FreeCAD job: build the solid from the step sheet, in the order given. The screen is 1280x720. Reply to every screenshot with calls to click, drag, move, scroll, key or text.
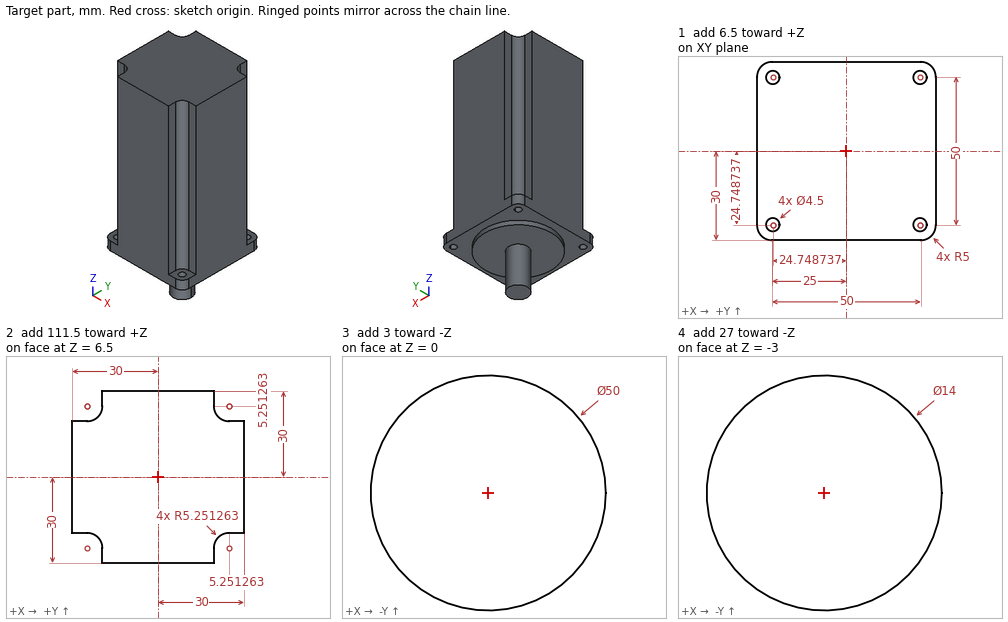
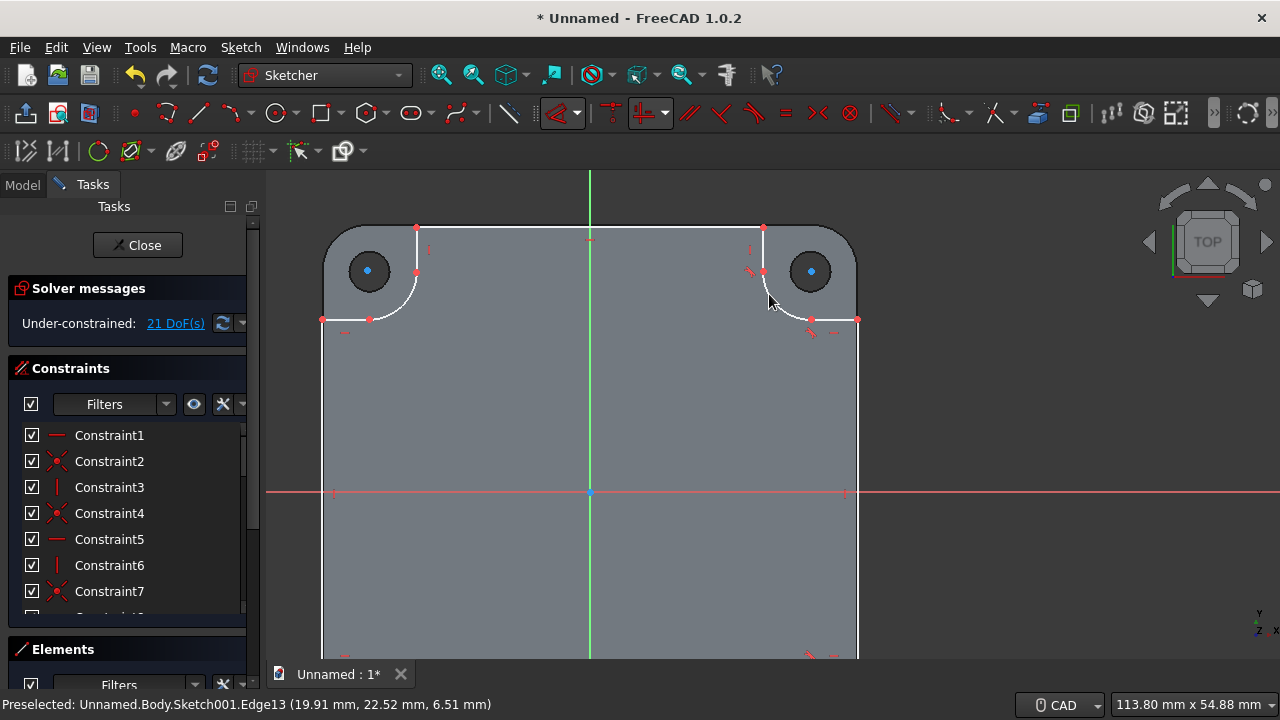
click(417, 241)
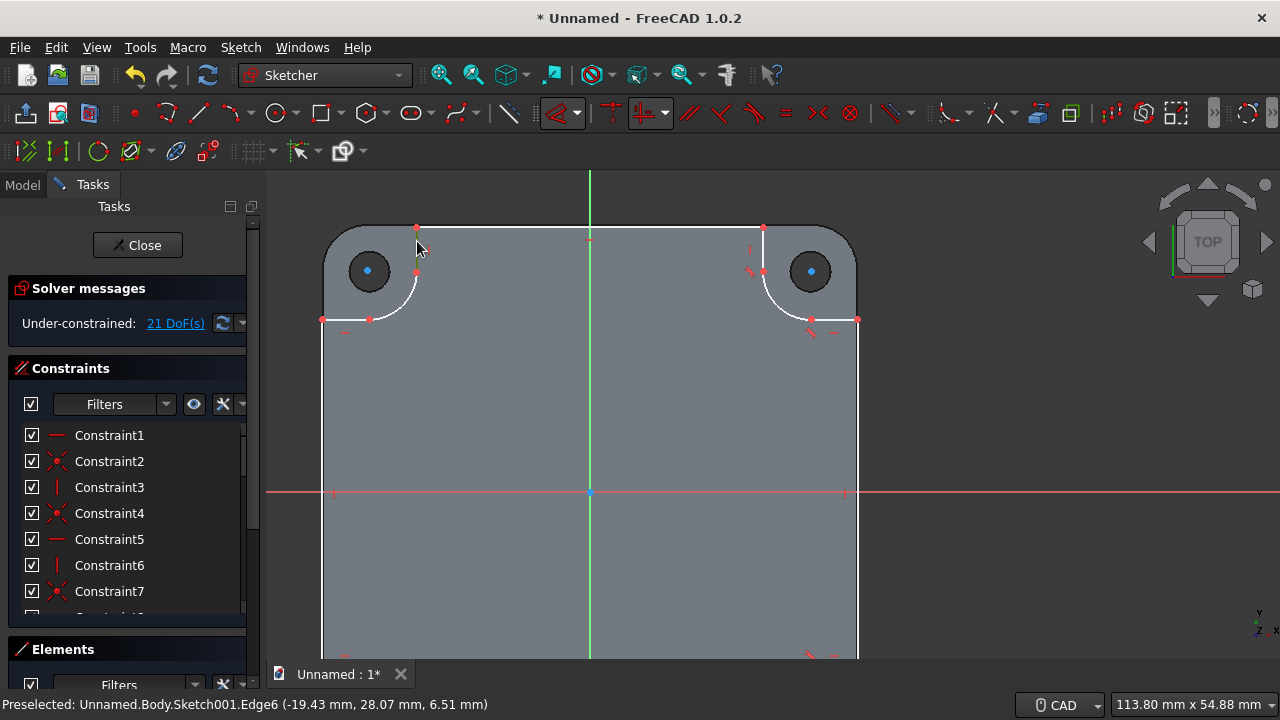
click(391, 314)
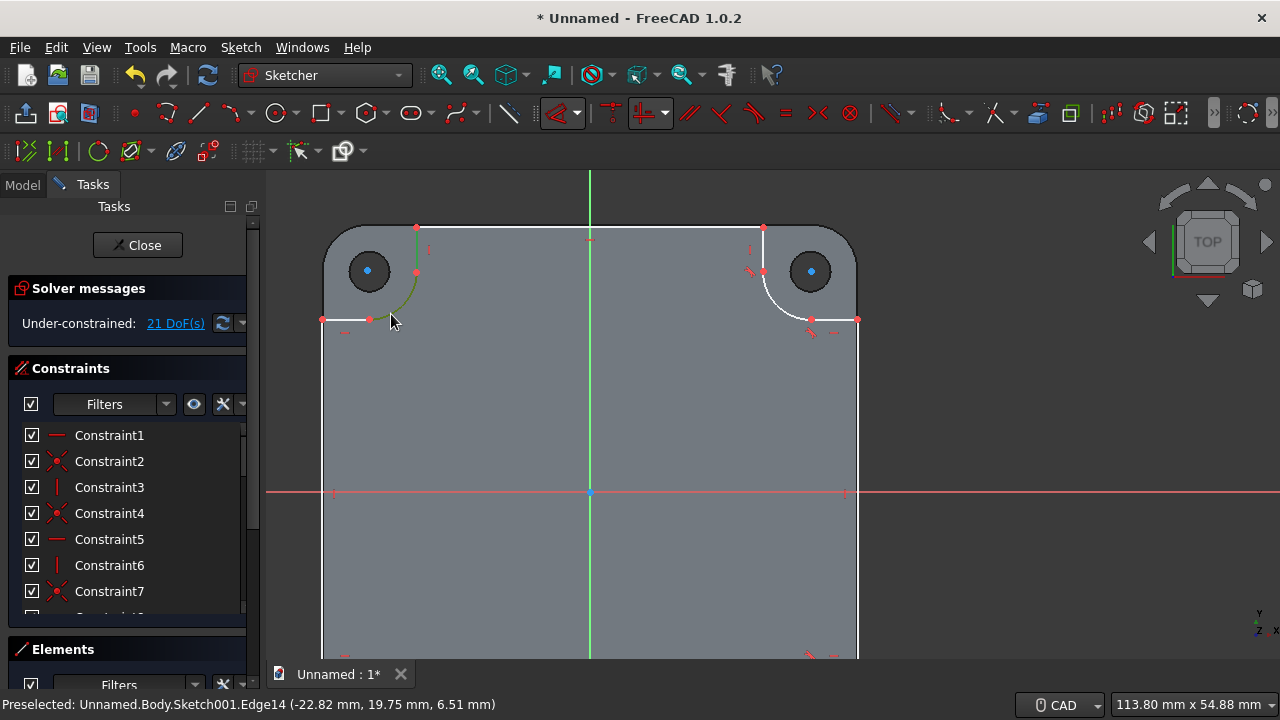
key(t)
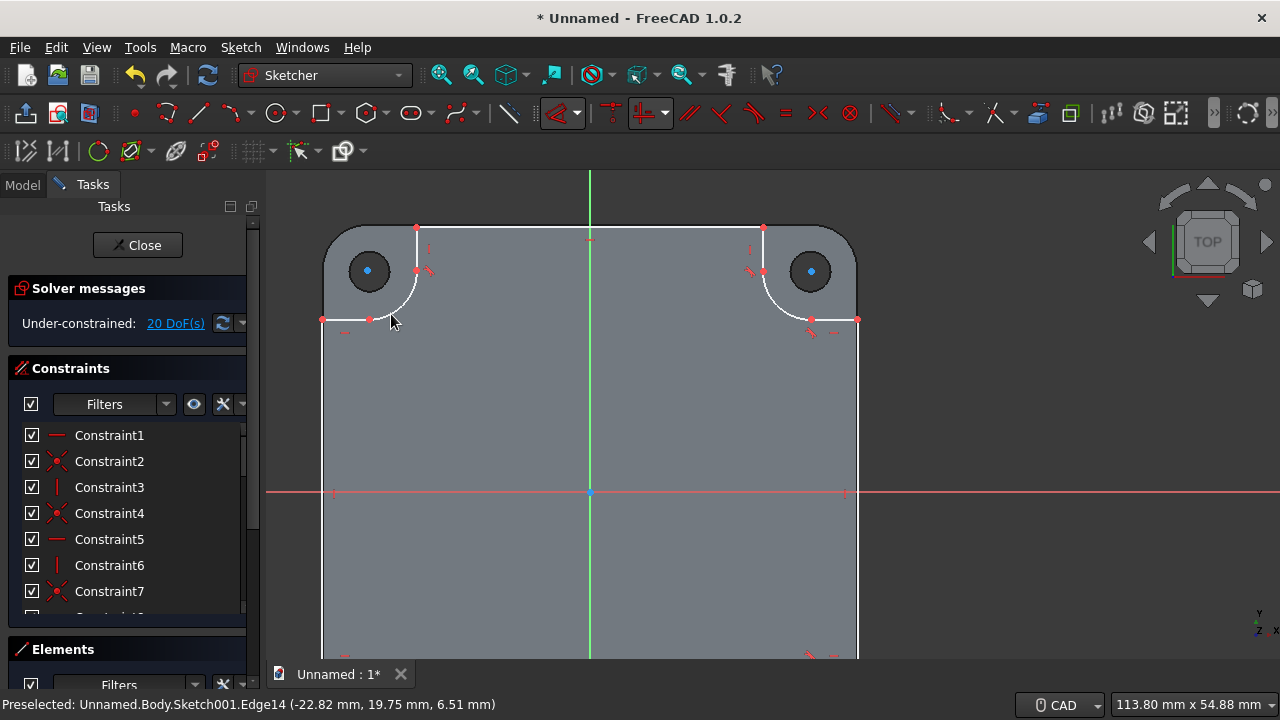
click(355, 320)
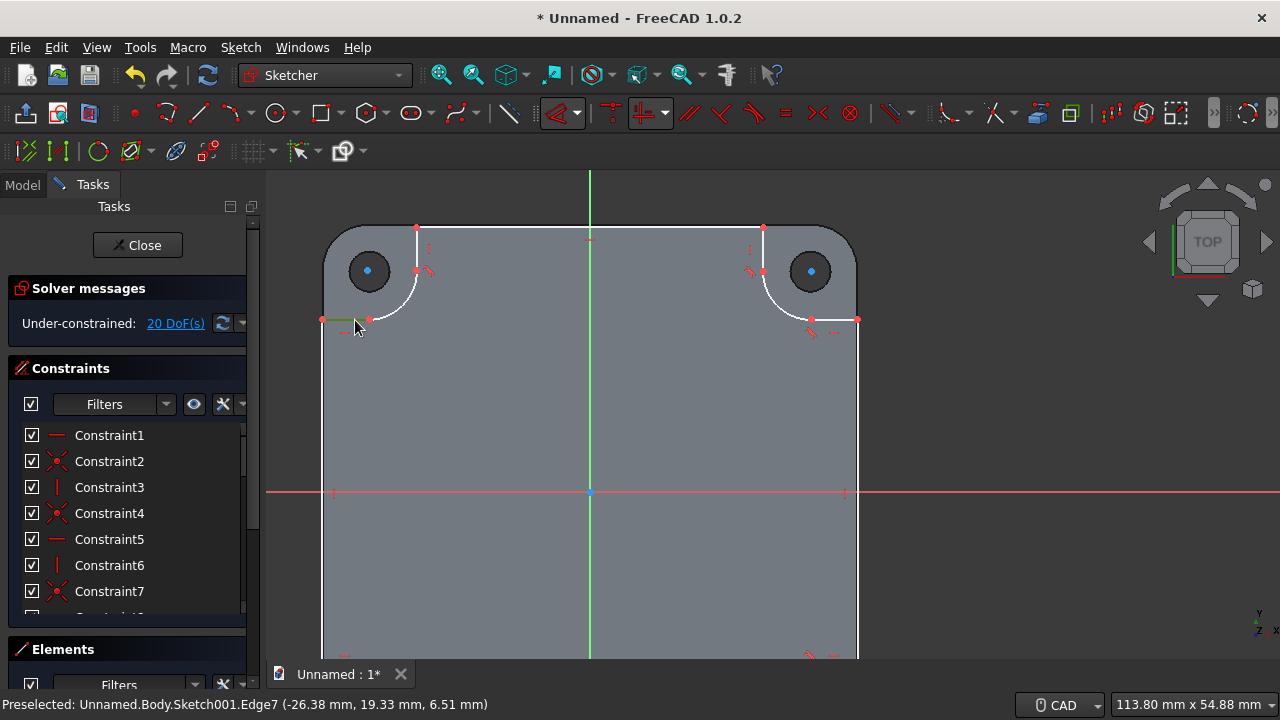
click(391, 314)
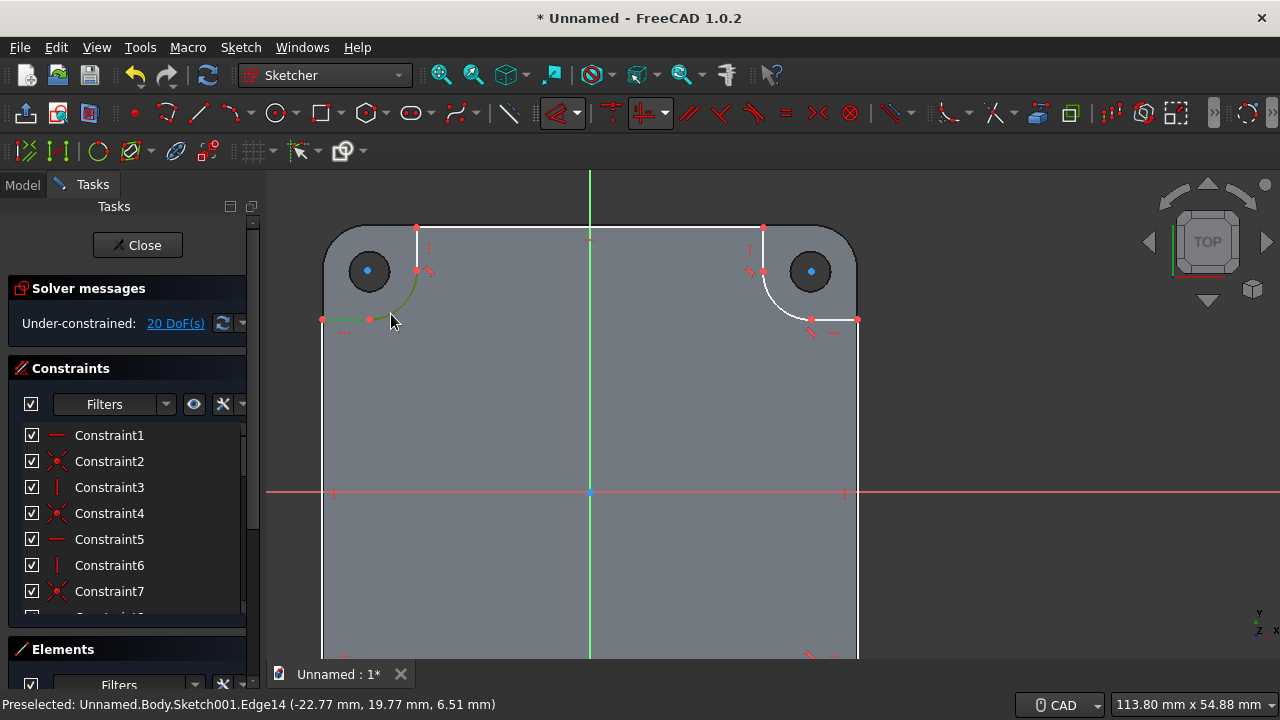
key(t)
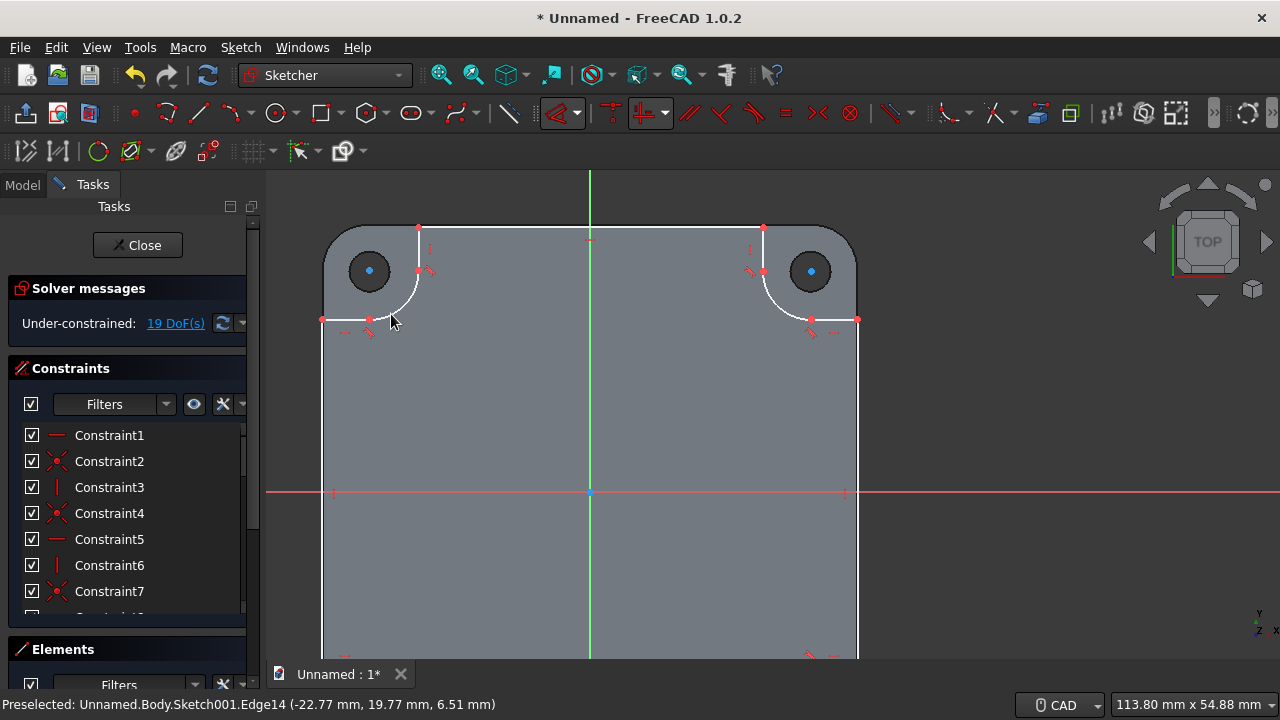
scroll(844, 320, down, 3)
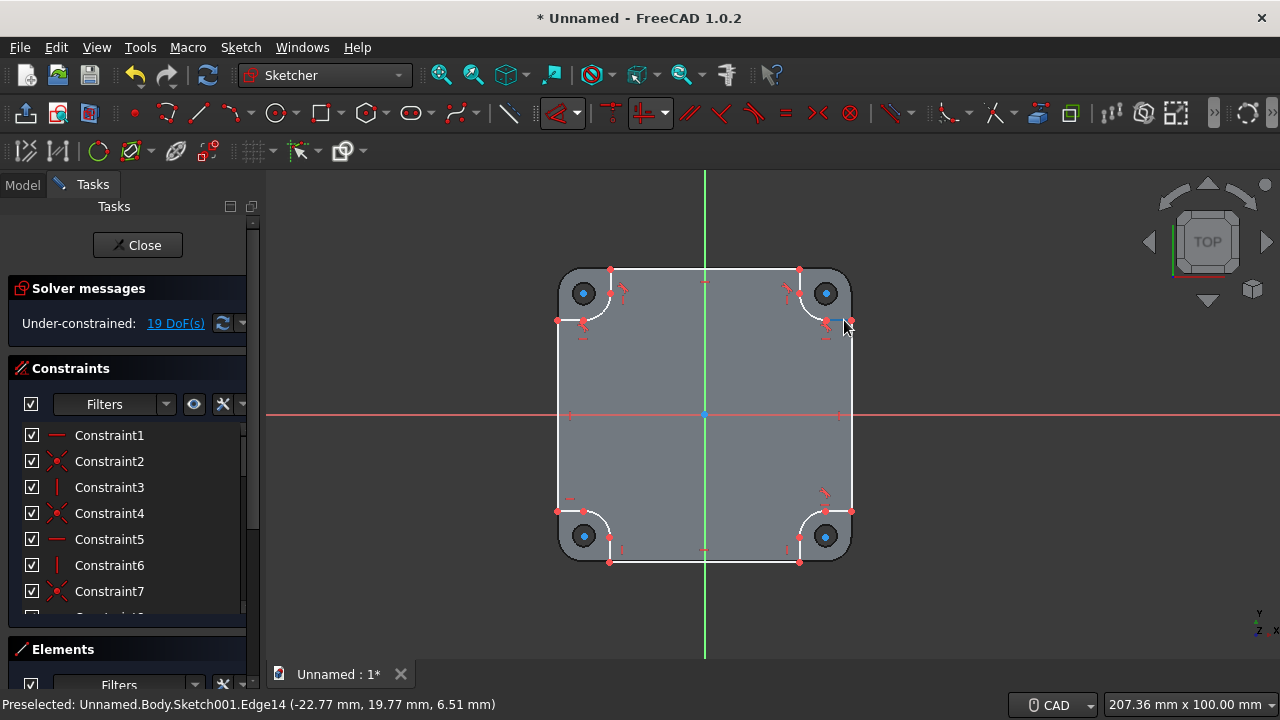
scroll(566, 511, up, 3)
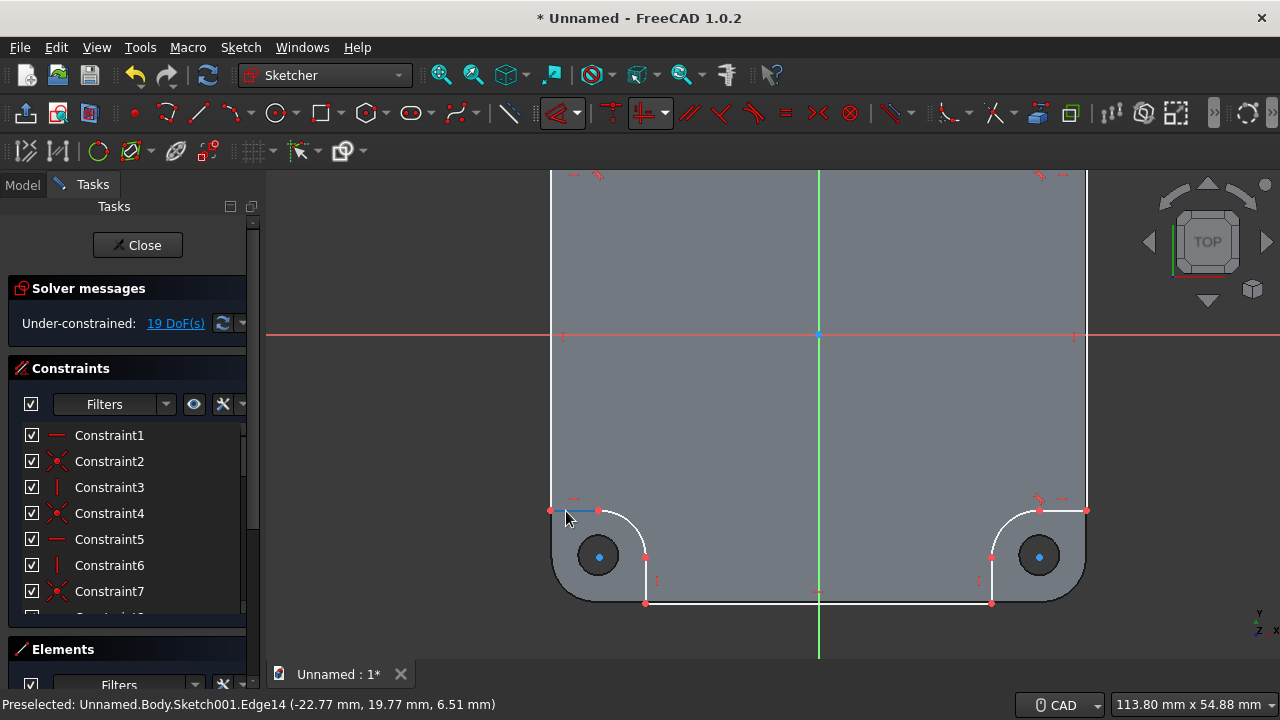
click(565, 511)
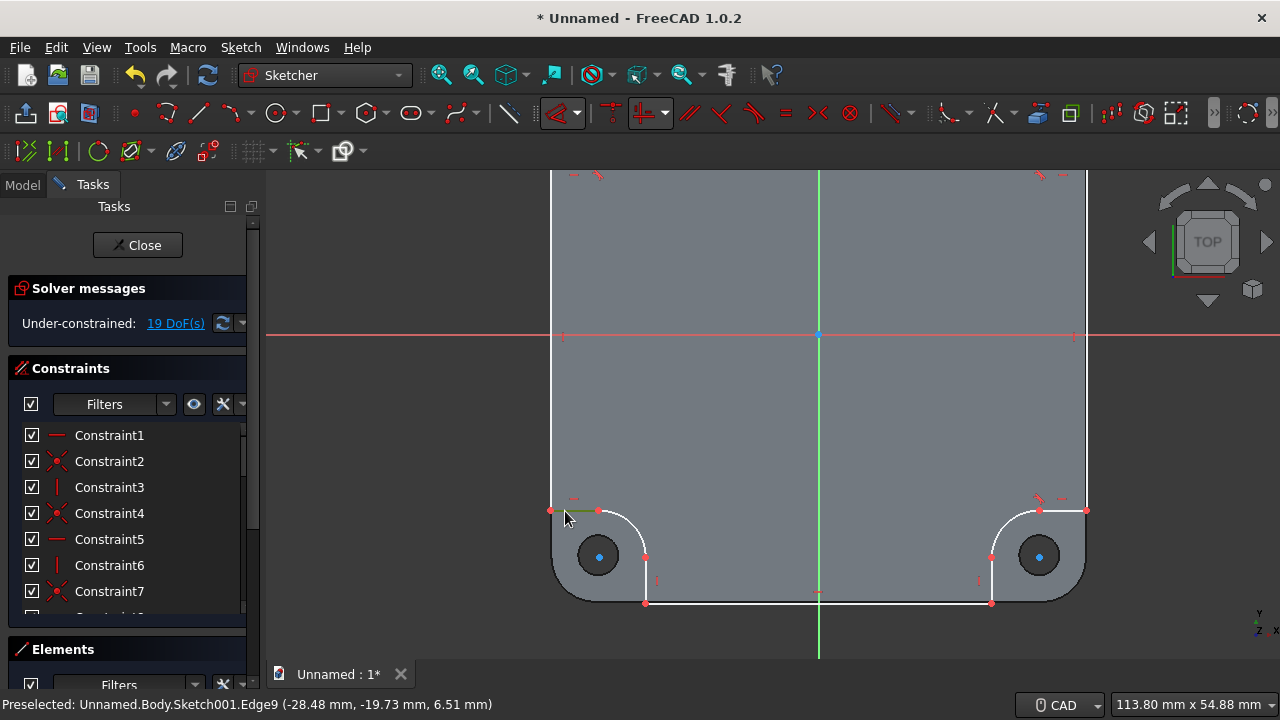
click(641, 536)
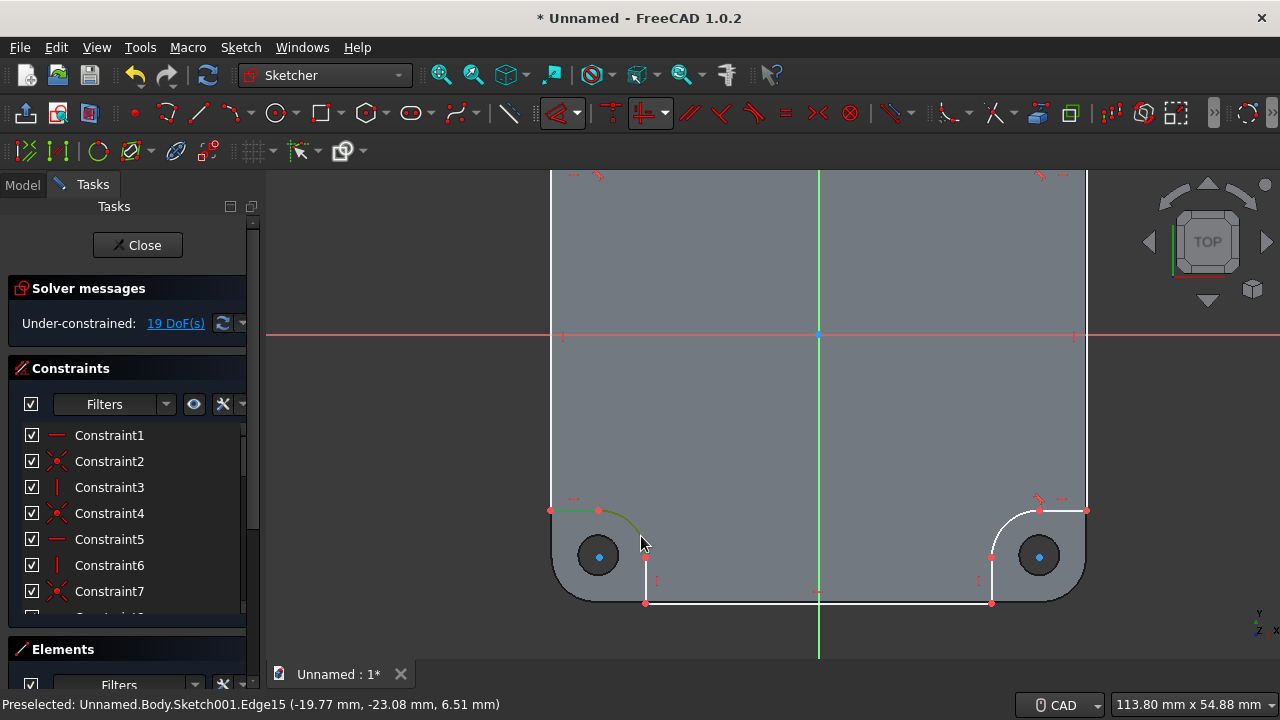
key(t)